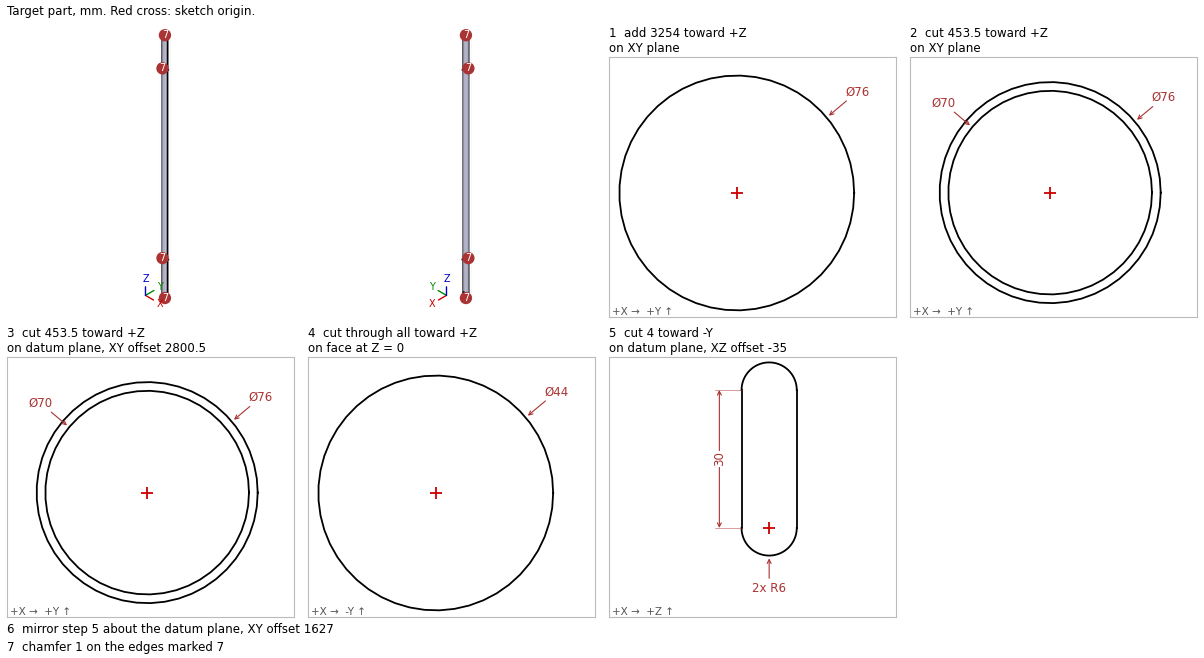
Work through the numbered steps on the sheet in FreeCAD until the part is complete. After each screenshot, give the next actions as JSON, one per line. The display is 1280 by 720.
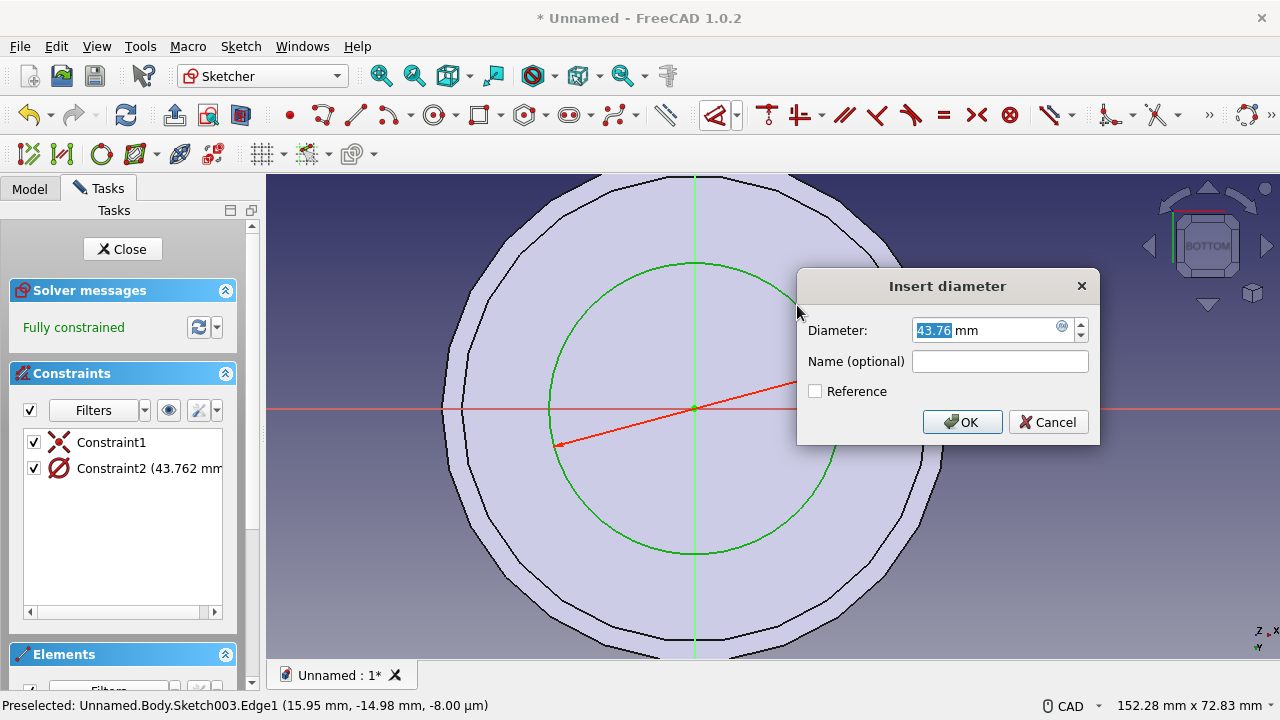
{"action": "type", "text": "44"}
{"action": "key", "text": "Return"}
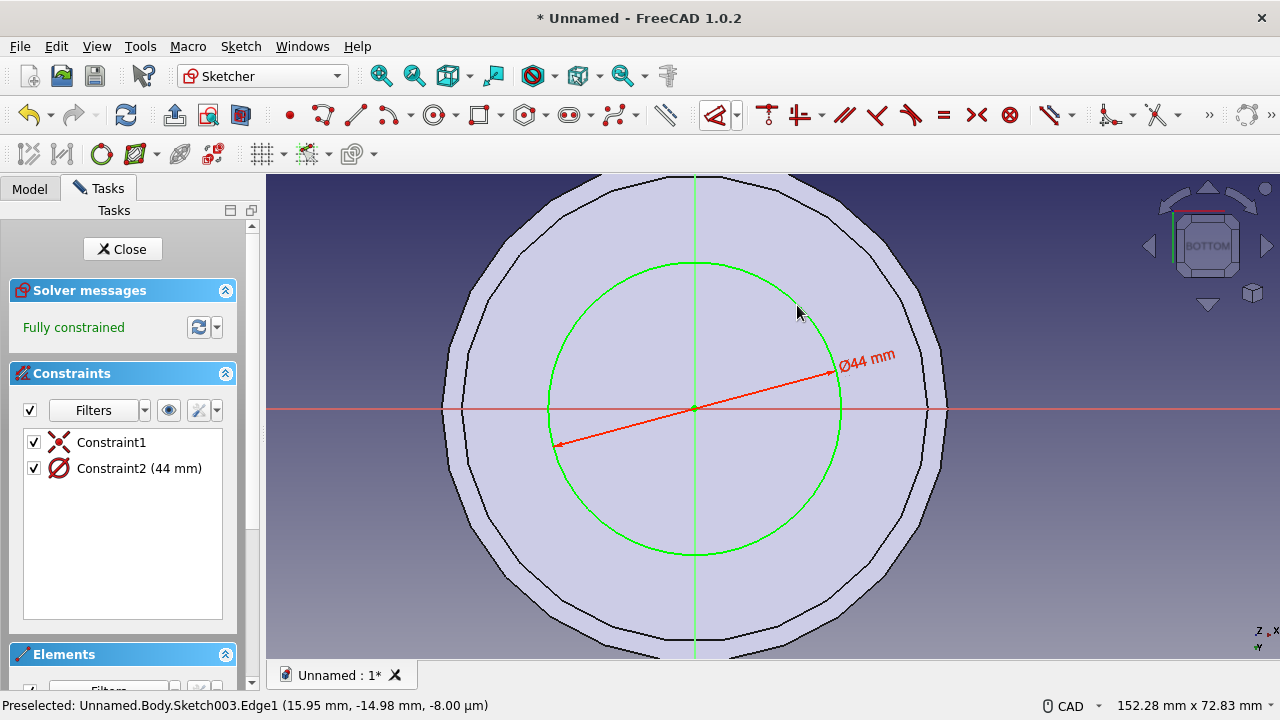
{"action": "left_click", "coordinate": [123, 249]}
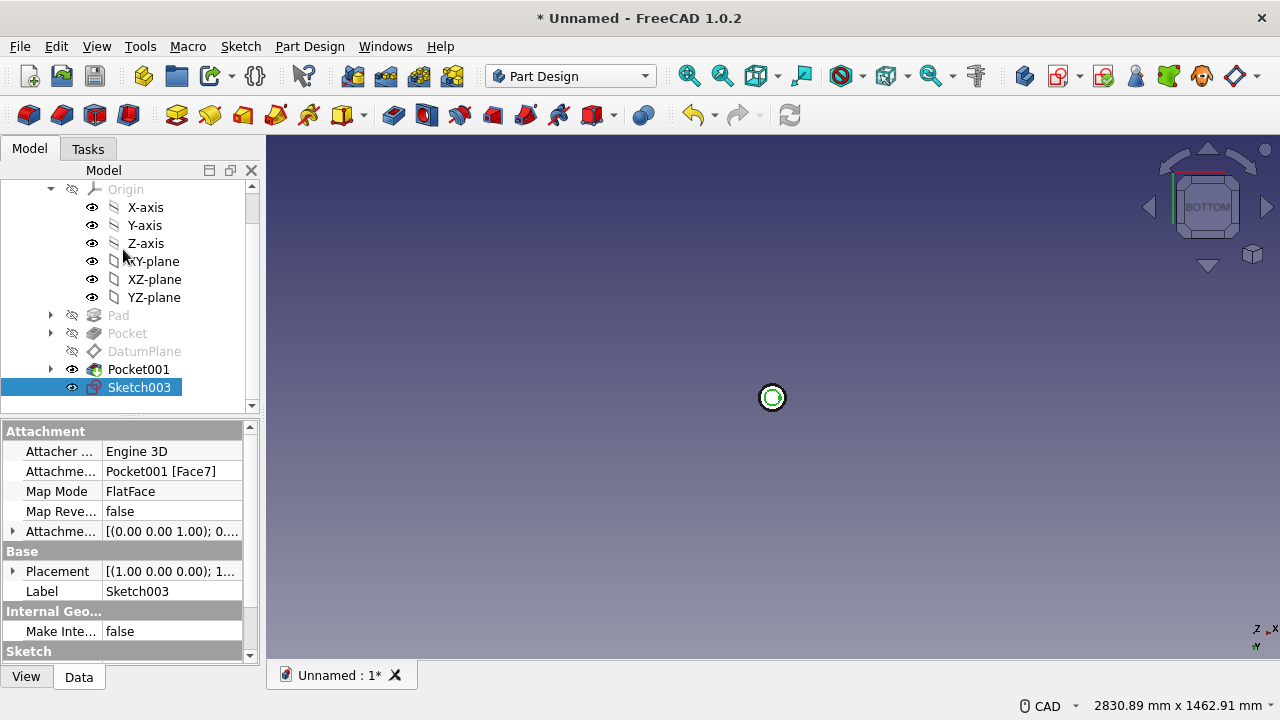
{"action": "left_click", "coordinate": [394, 116]}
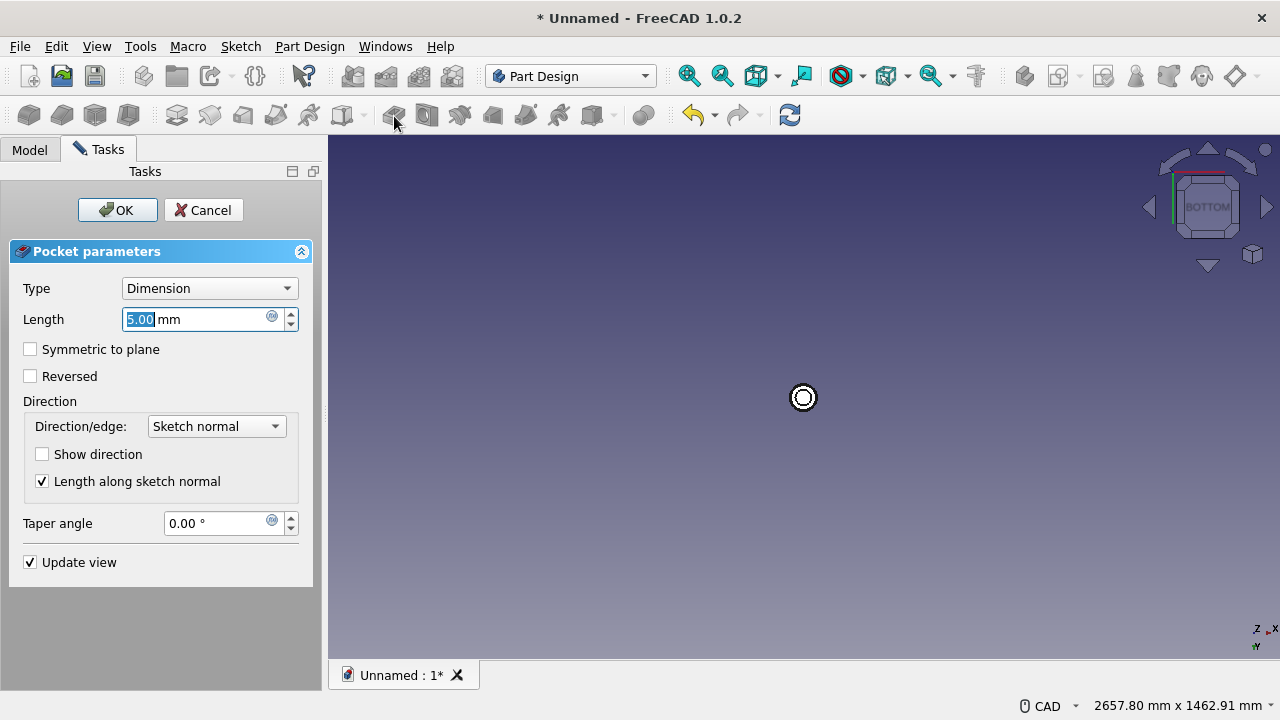
{"action": "left_click", "coordinate": [210, 288]}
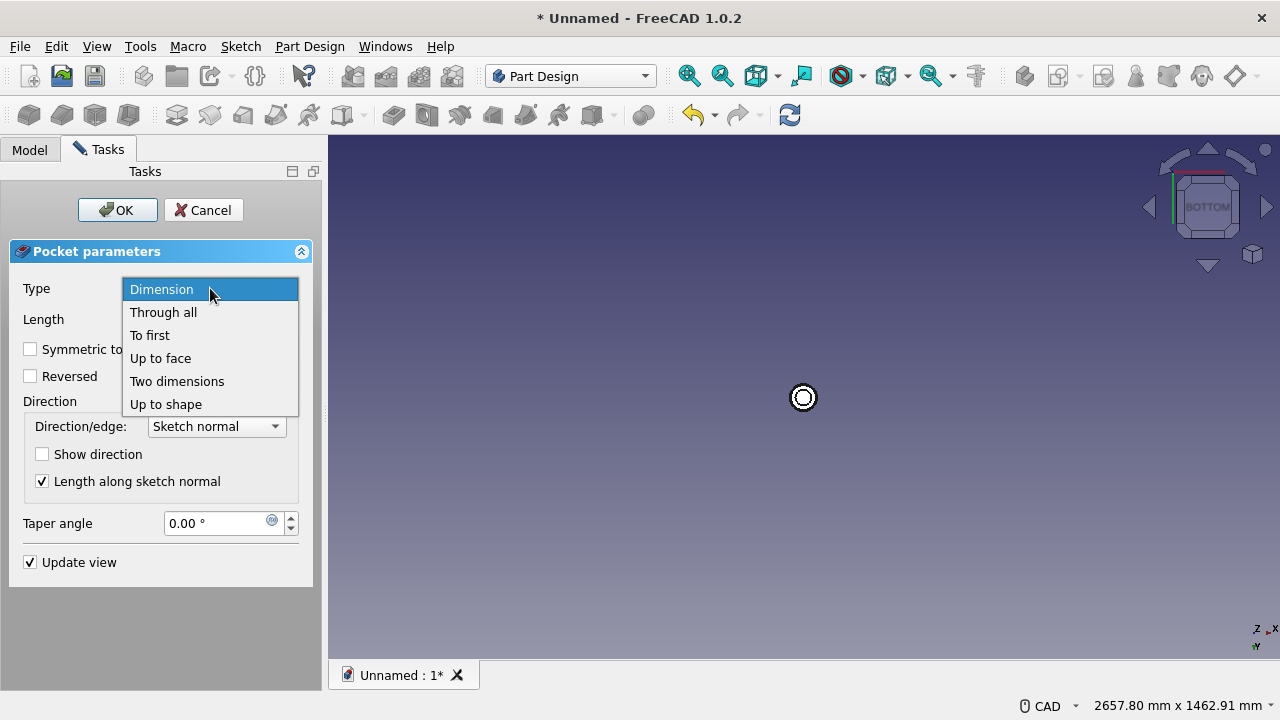
{"action": "left_click", "coordinate": [208, 312]}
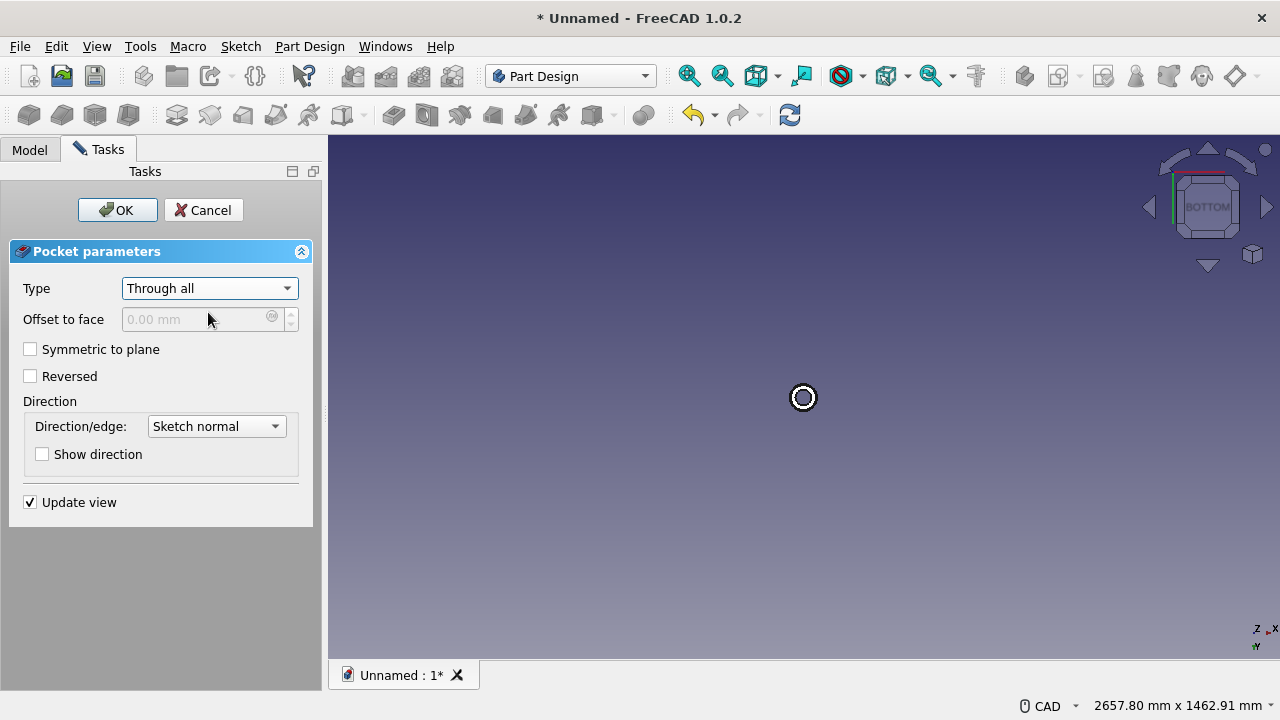
{"action": "left_click", "coordinate": [118, 210]}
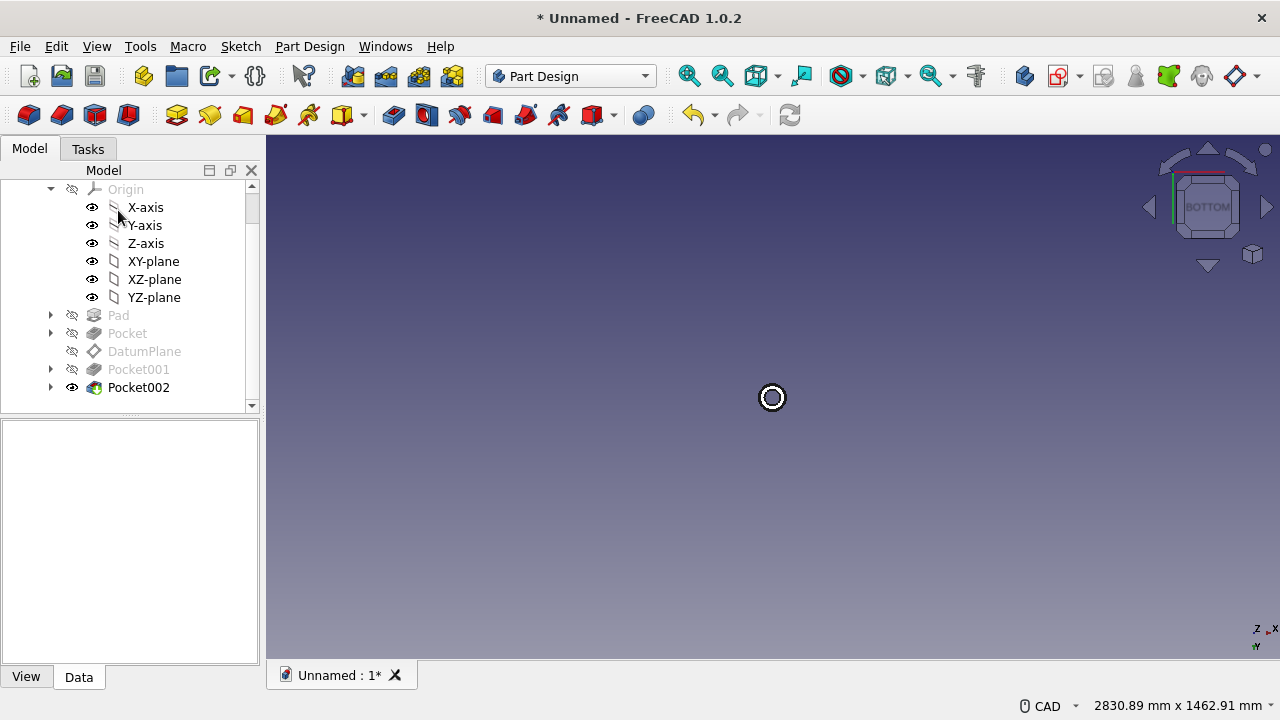
{"action": "left_click", "coordinate": [690, 76]}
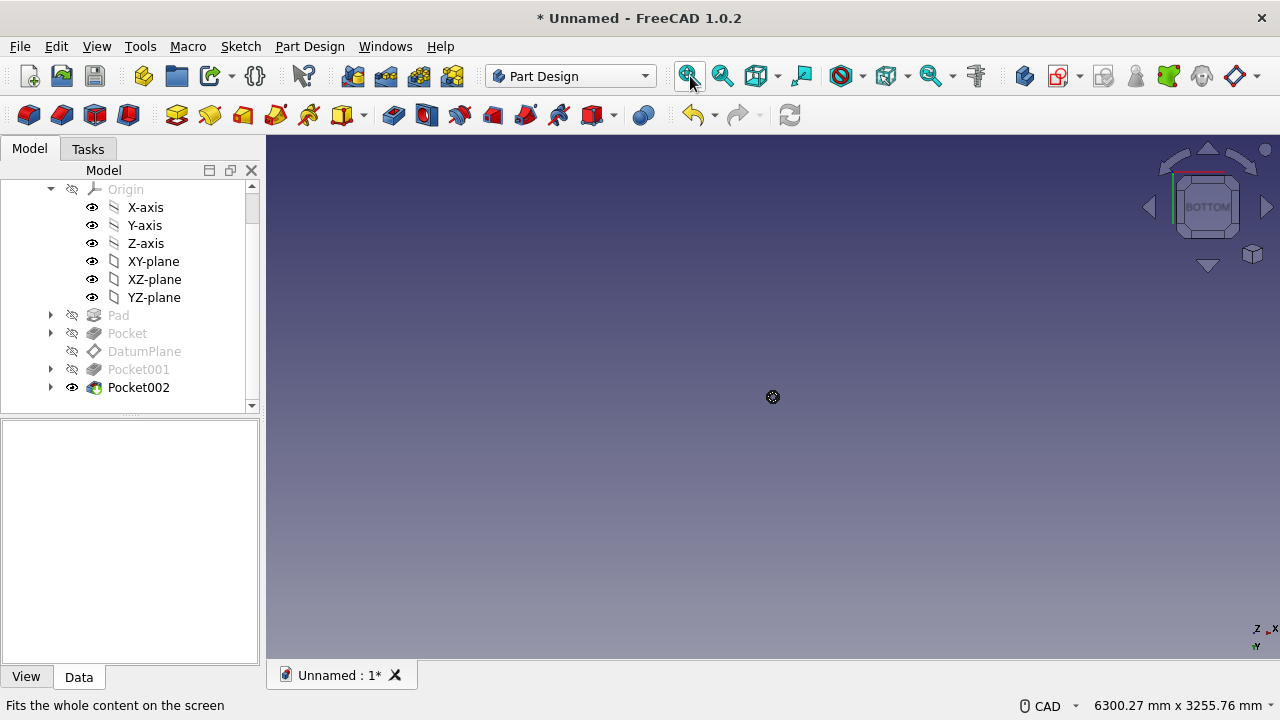
{"action": "left_click", "coordinate": [137, 279]}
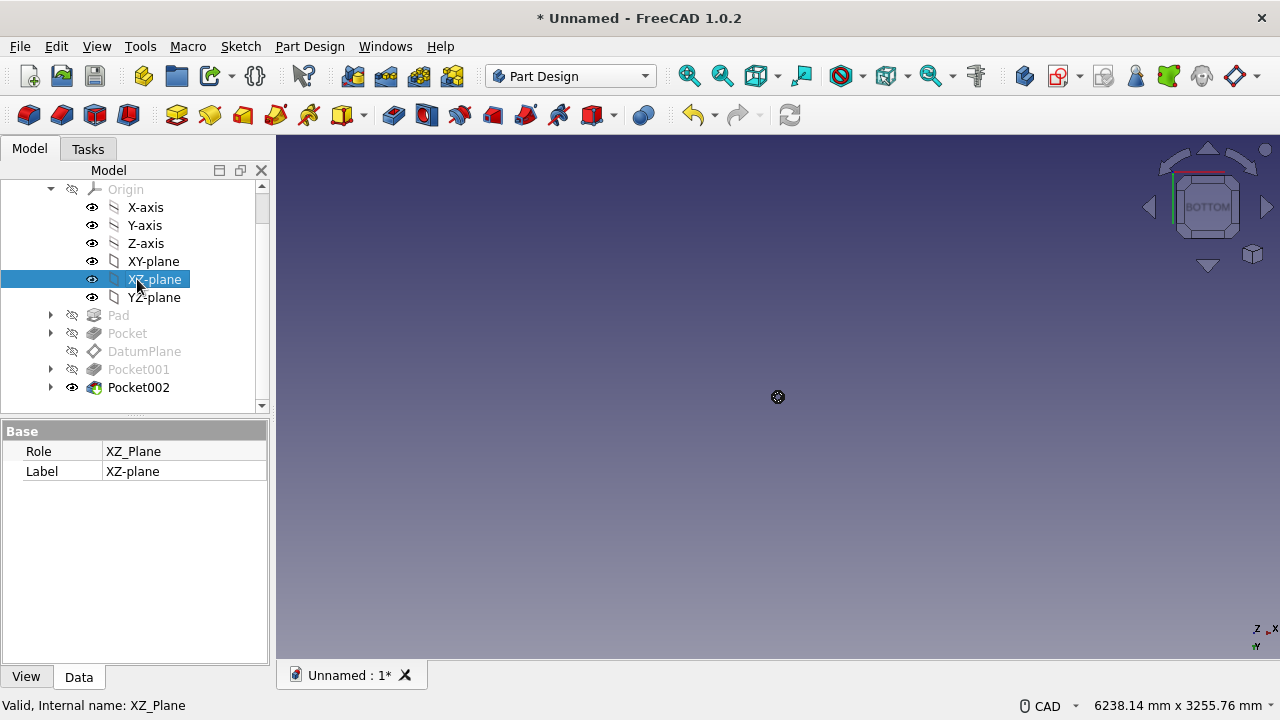
{"action": "left_click", "coordinate": [1234, 76]}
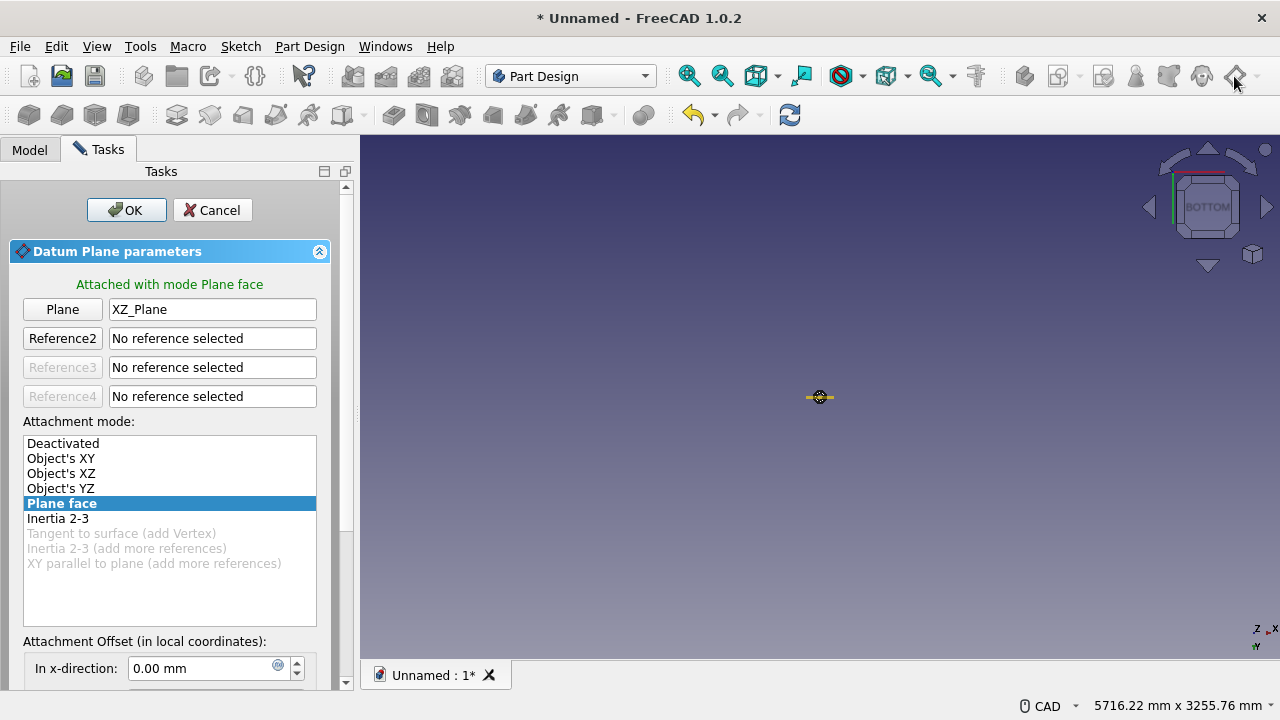
{"action": "scroll", "coordinate": [346, 436], "scroll_direction": "down", "scroll_amount": 2}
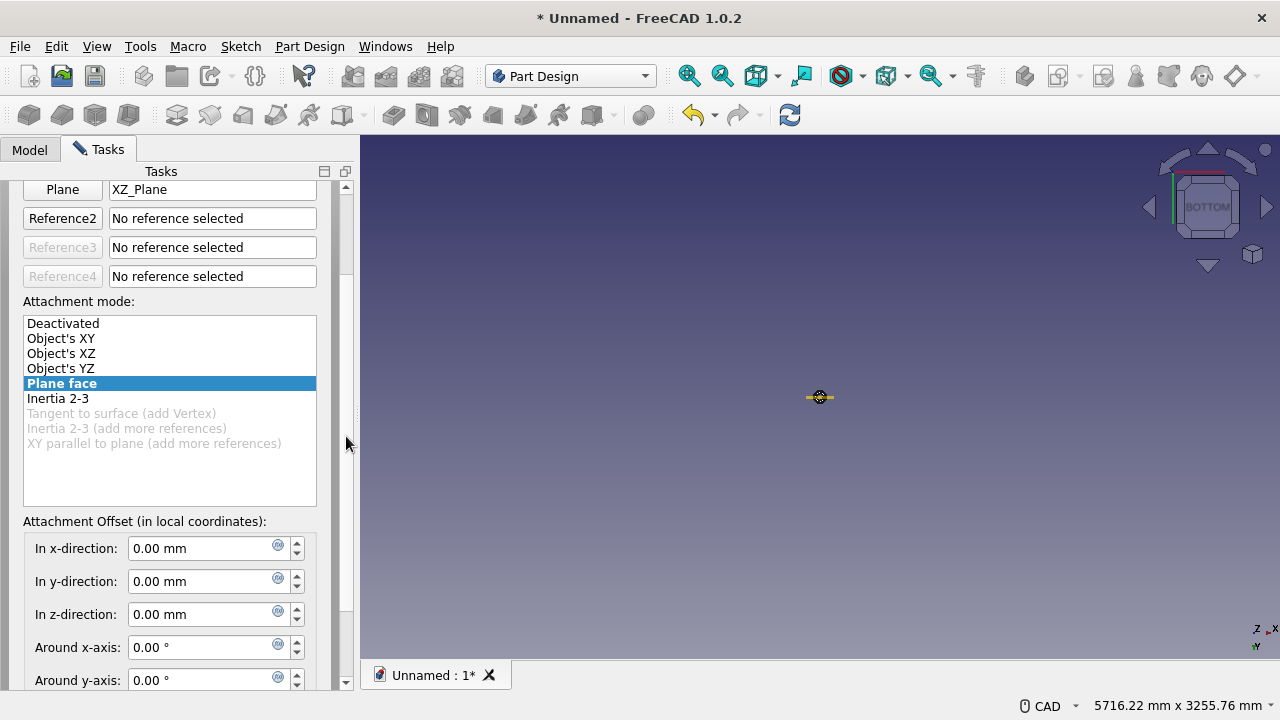
{"action": "triple_click", "coordinate": [210, 614]}